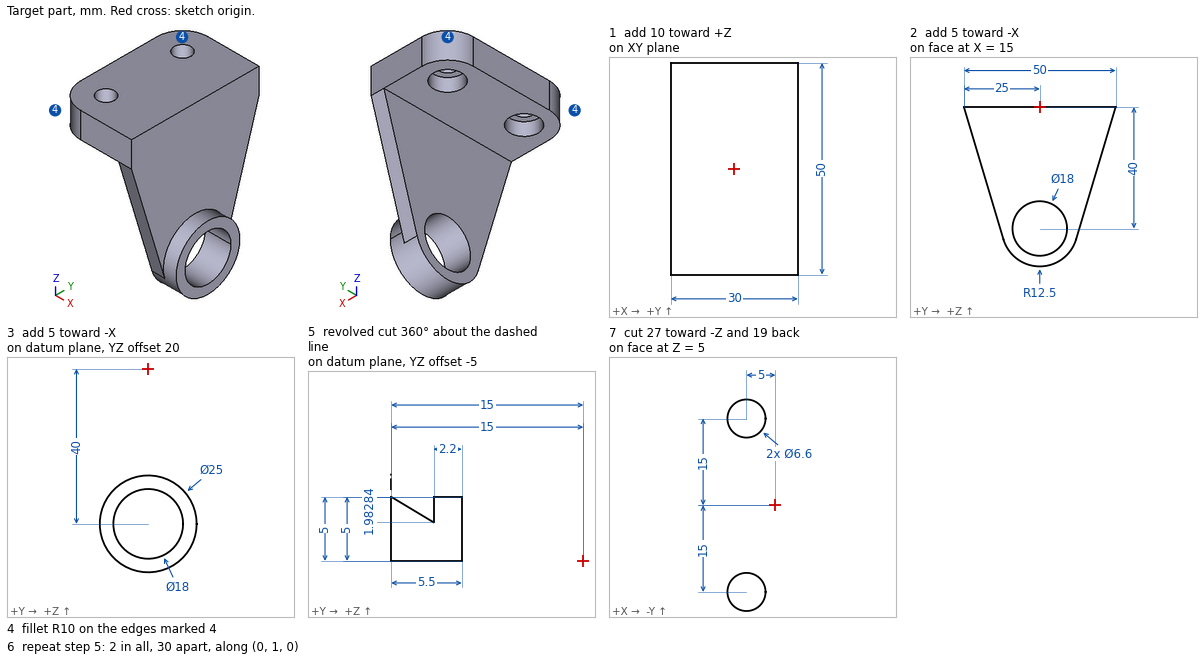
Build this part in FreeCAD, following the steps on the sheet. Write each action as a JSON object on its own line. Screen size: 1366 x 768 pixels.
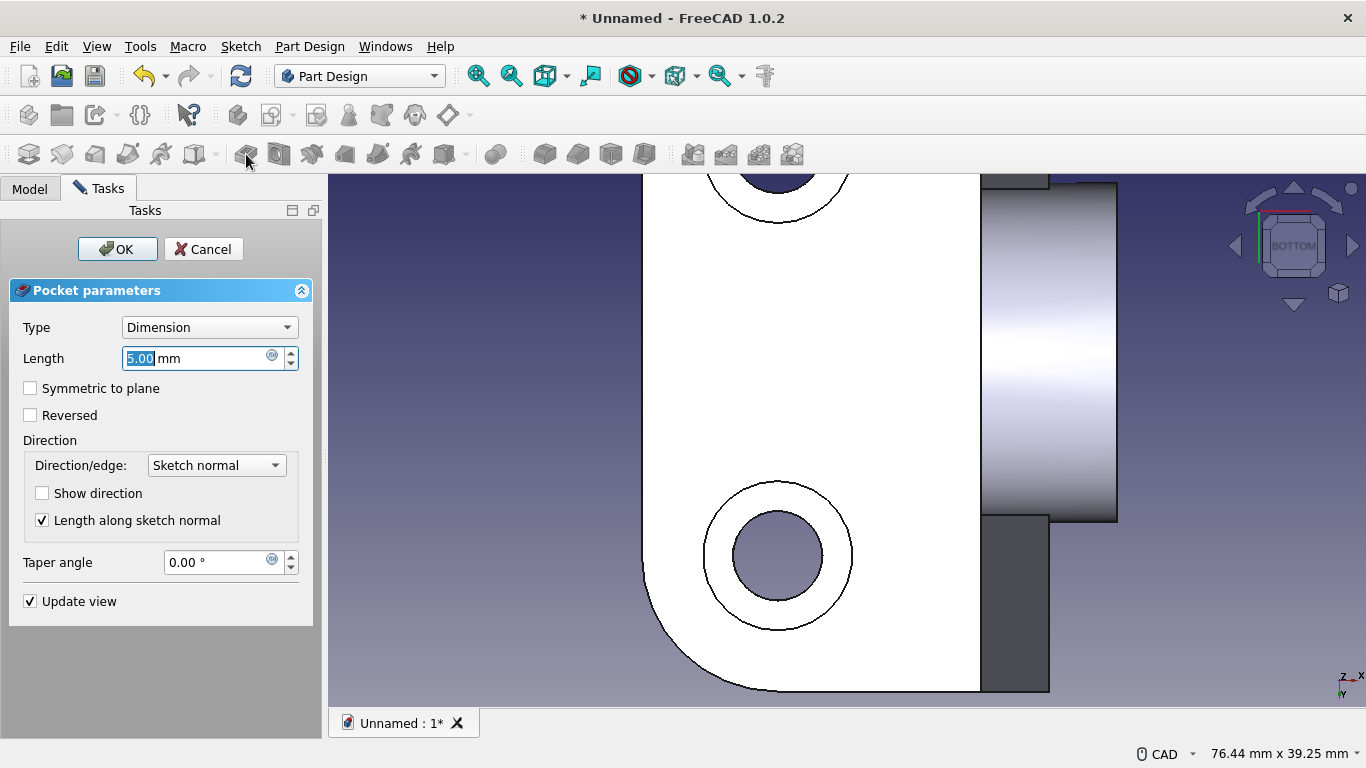
{"action": "left_click", "coordinate": [210, 328]}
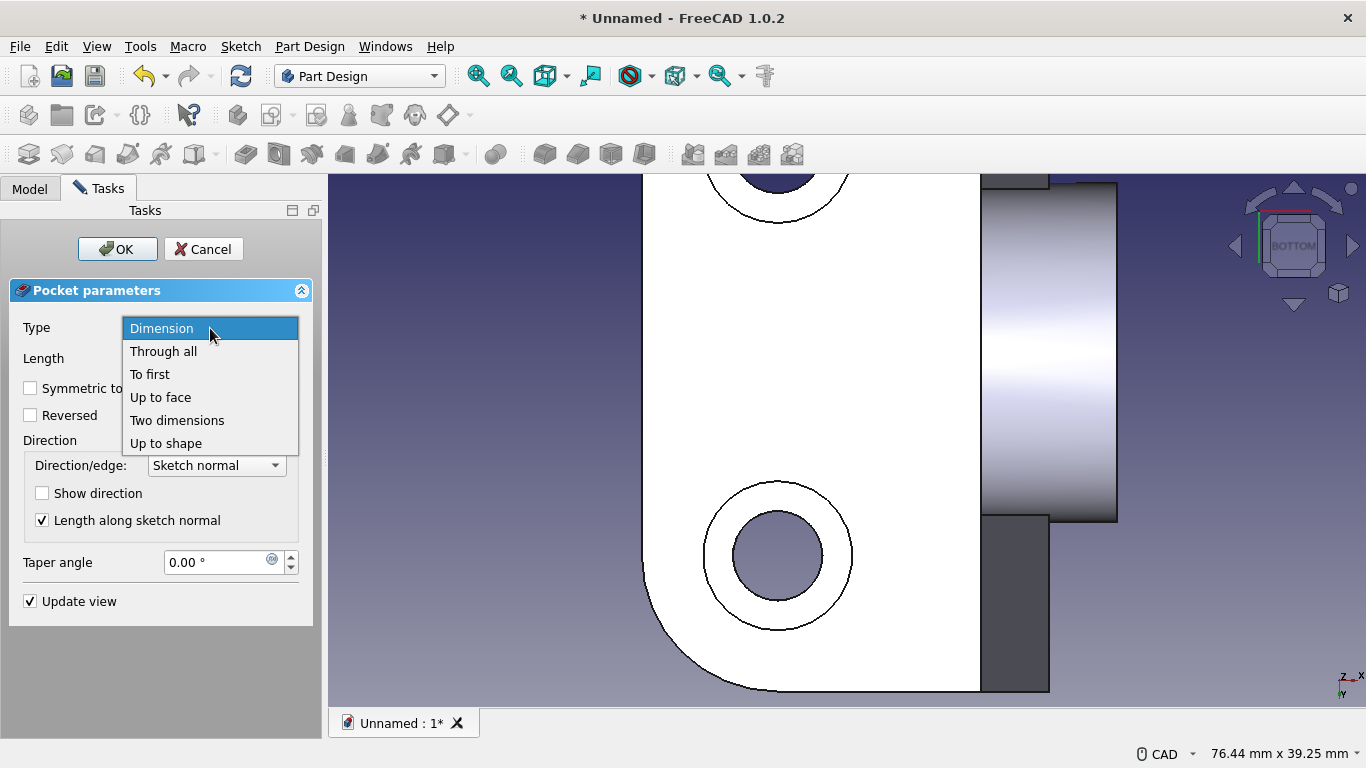
{"action": "left_click", "coordinate": [208, 420]}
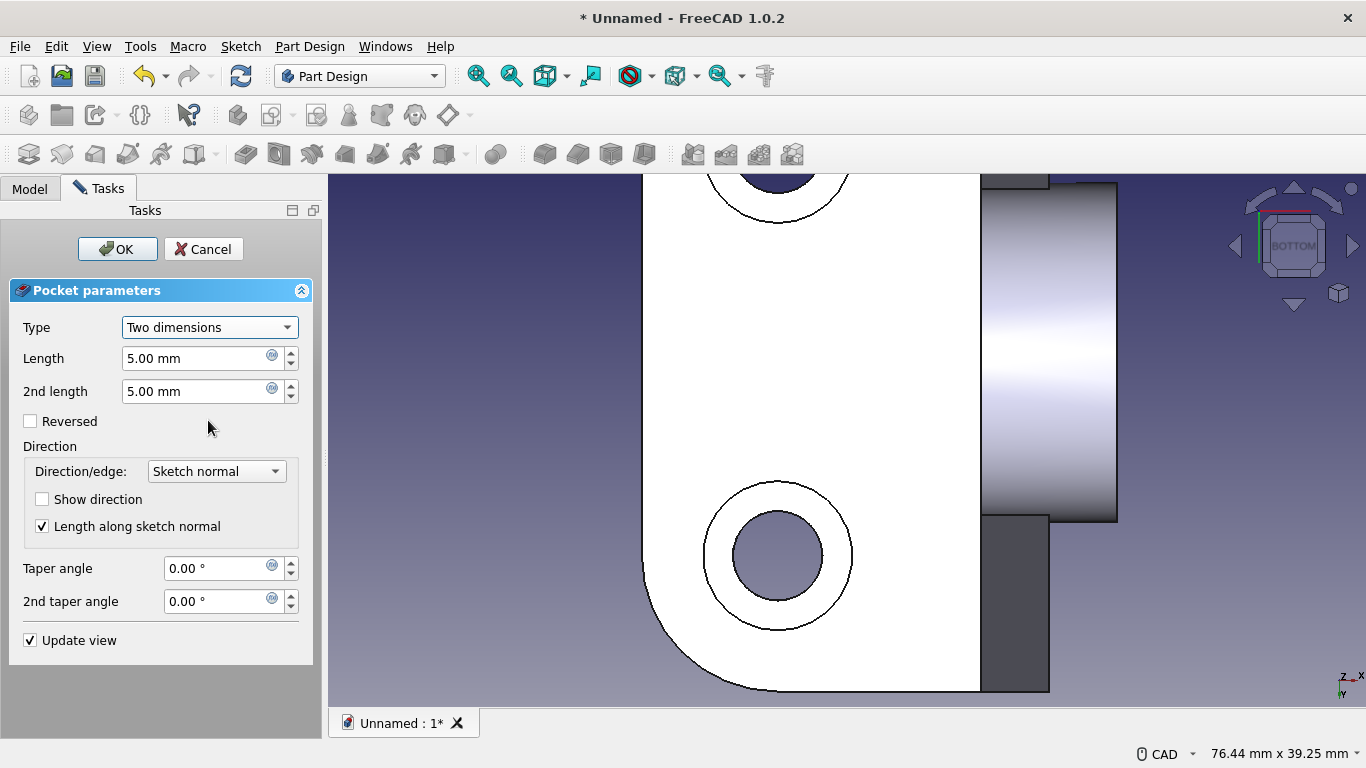
{"action": "triple_click", "coordinate": [204, 358]}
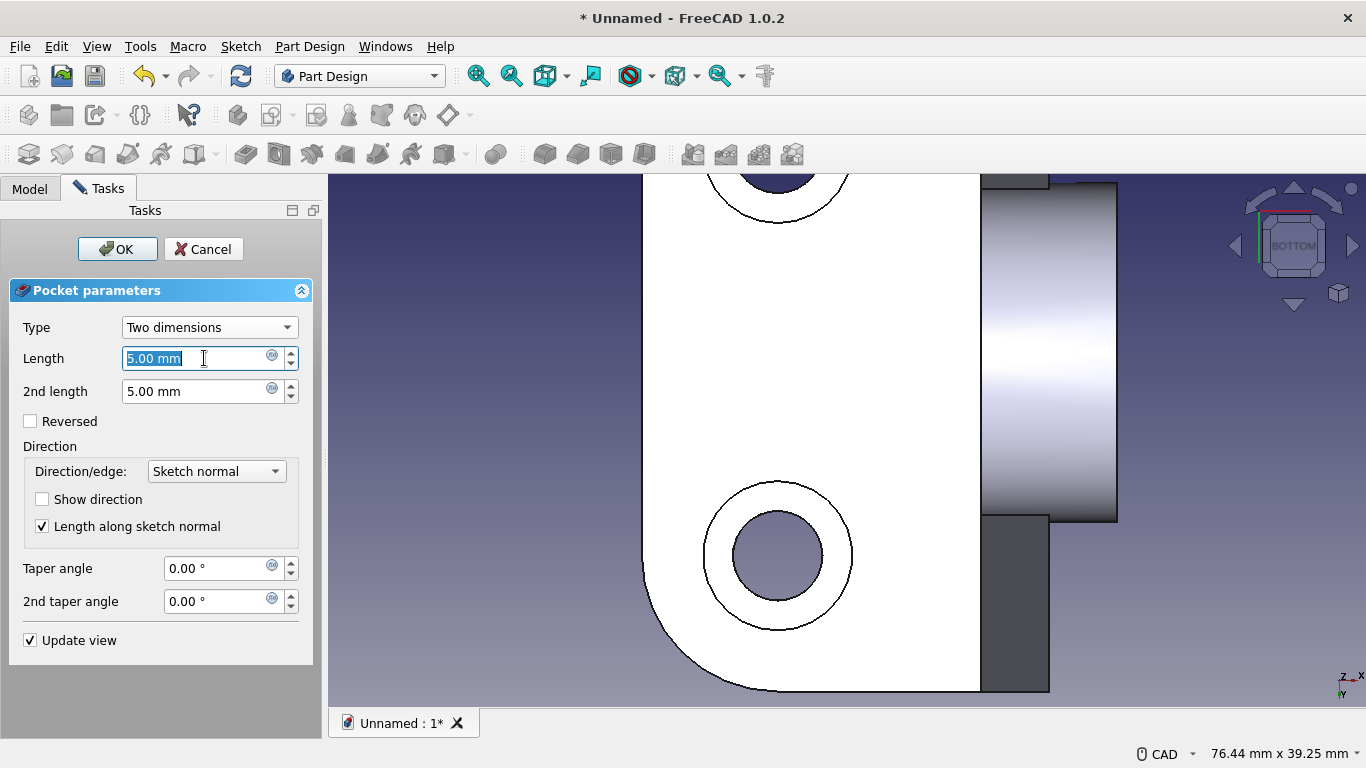
{"action": "type", "text": "27"}
{"action": "key", "text": "Tab"}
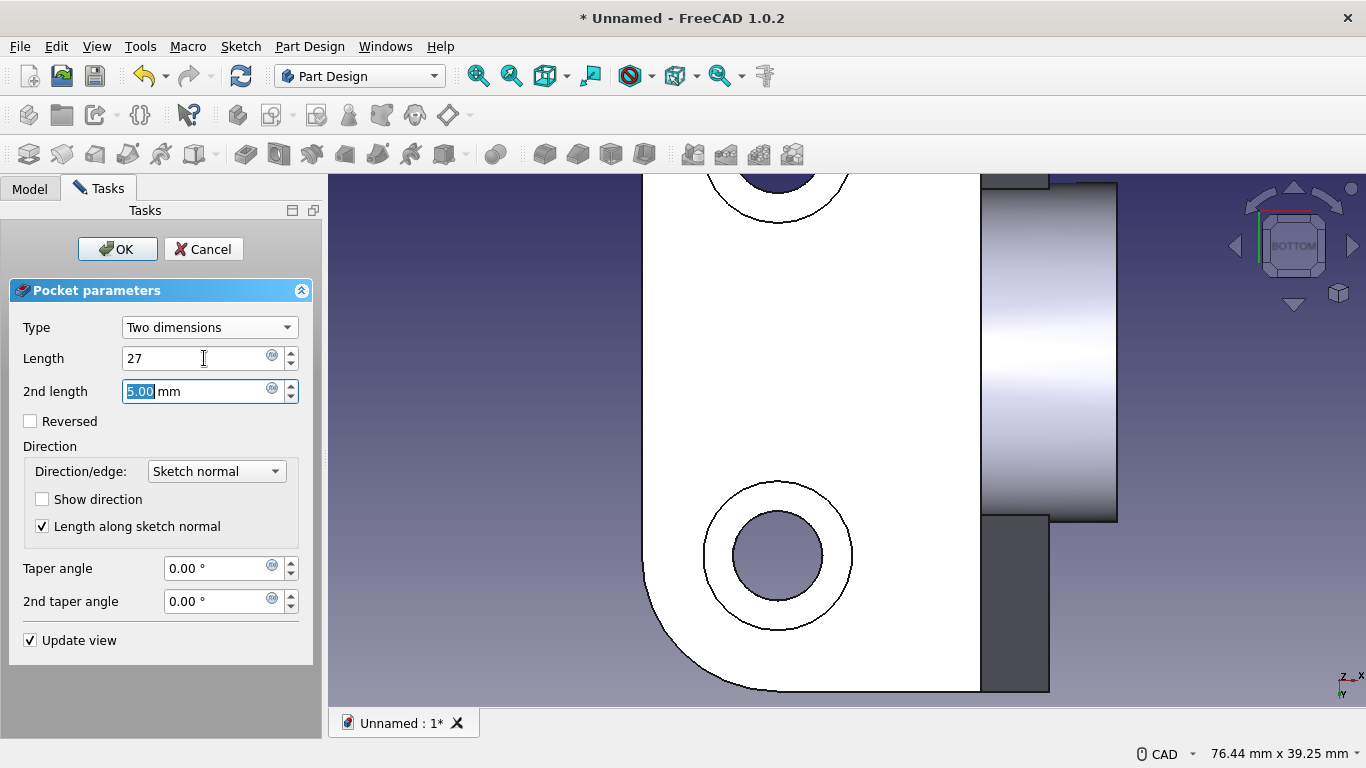
{"action": "type", "text": "19"}
{"action": "key", "text": "Tab"}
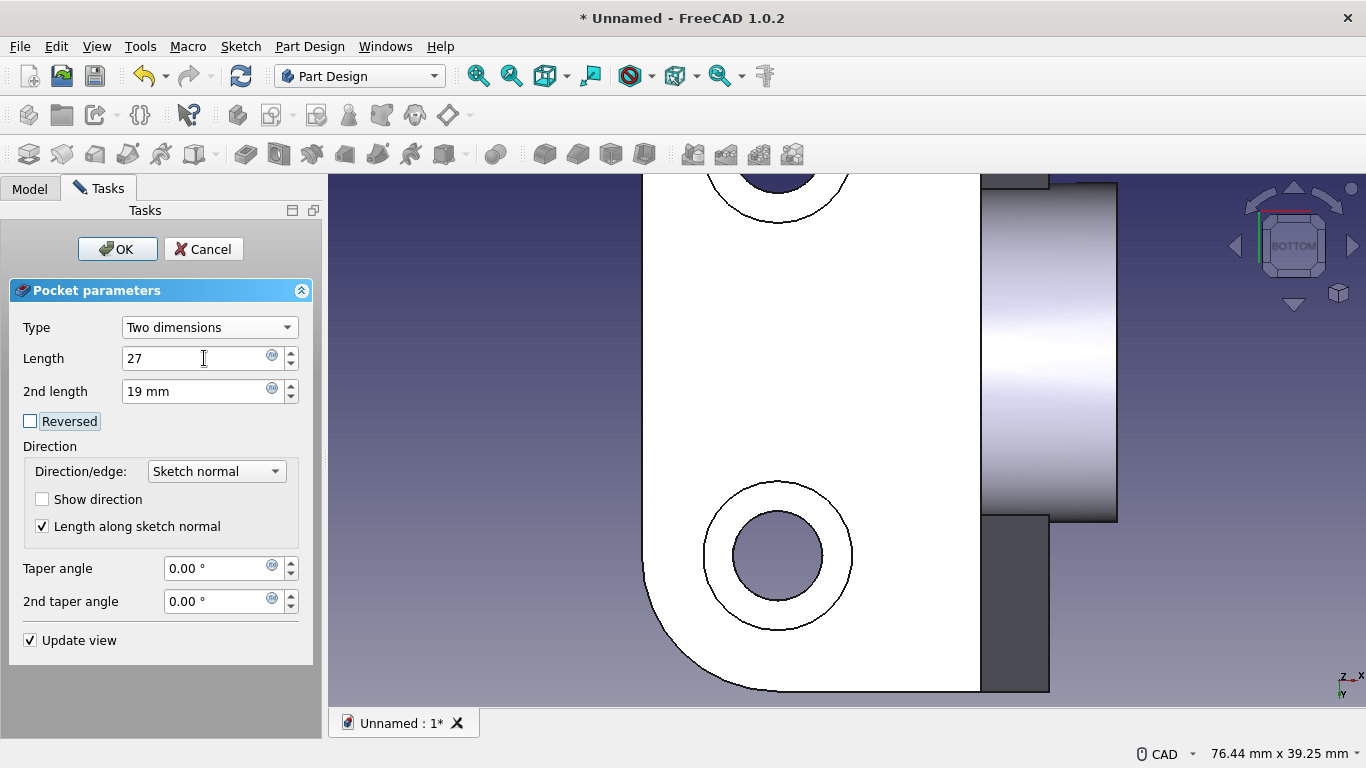
{"action": "left_click", "coordinate": [31, 421]}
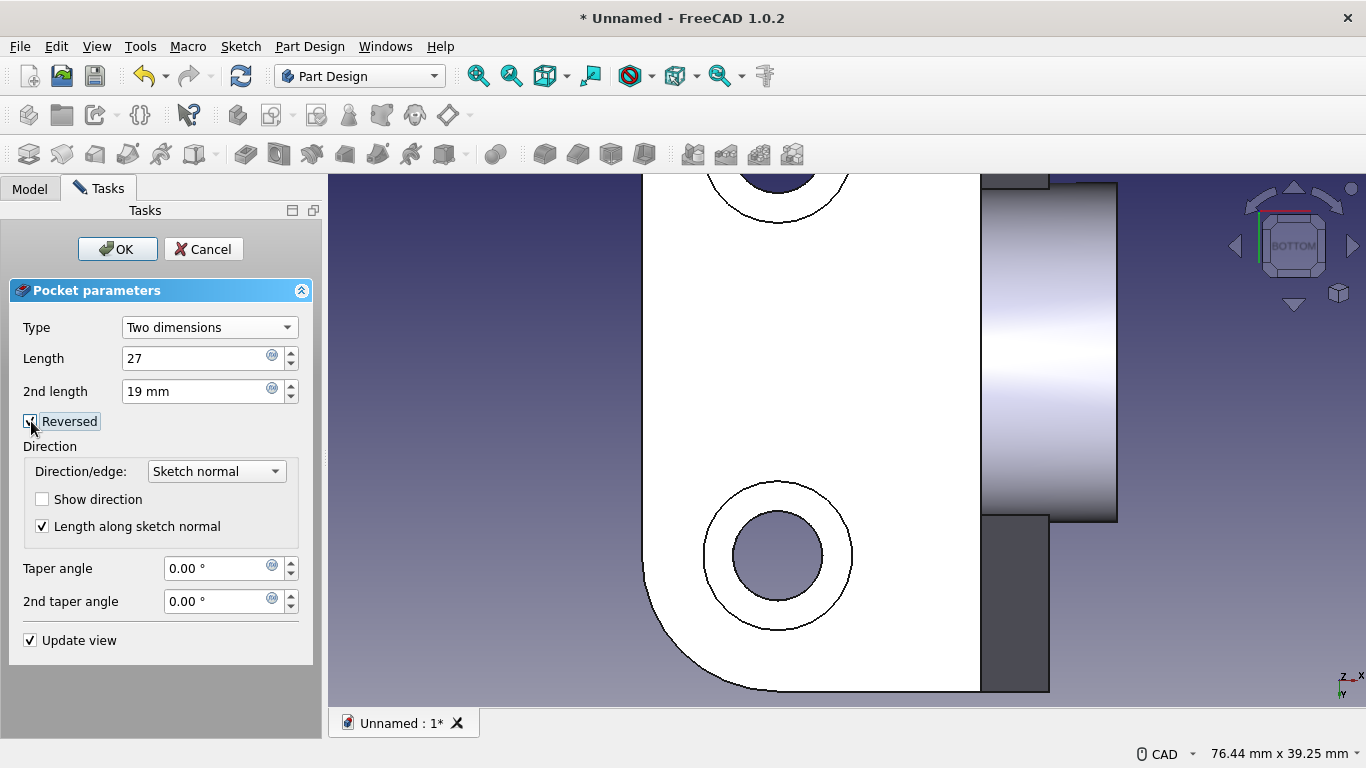
{"action": "left_click", "coordinate": [118, 249]}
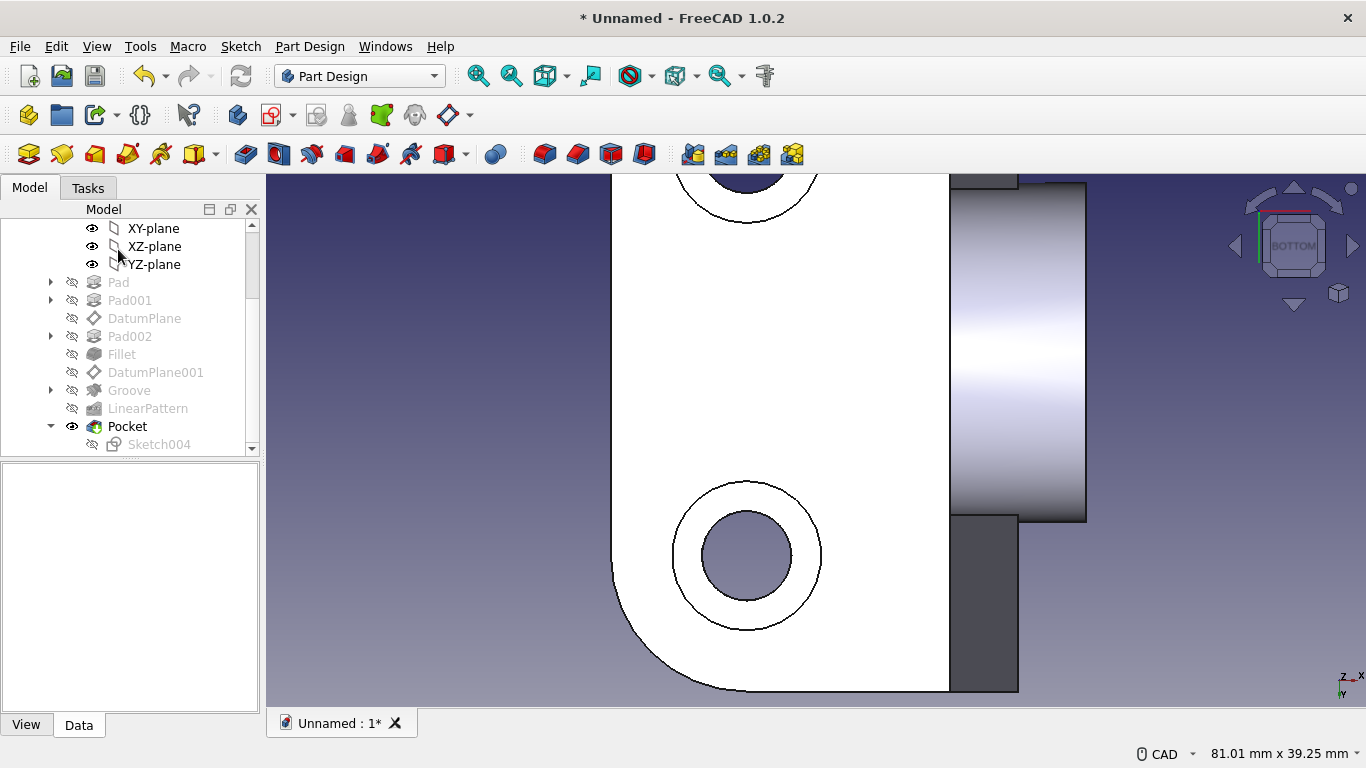
{"action": "key", "text": "0"}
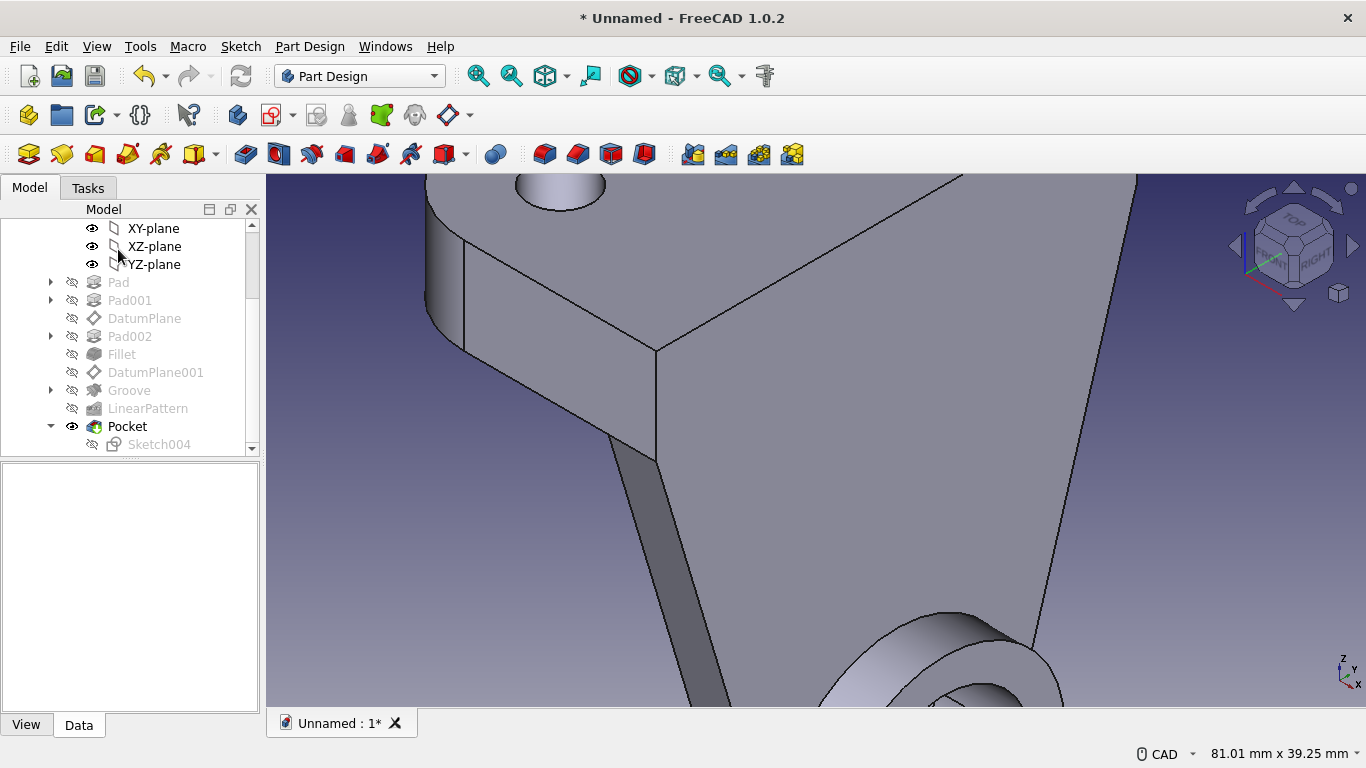
{"action": "left_click", "coordinate": [479, 76]}